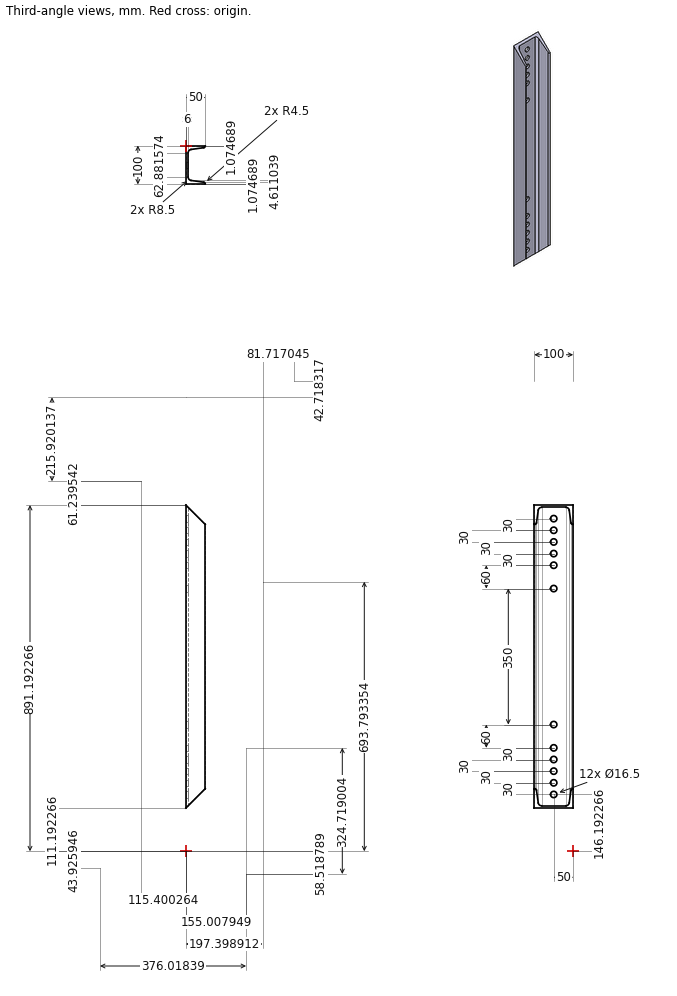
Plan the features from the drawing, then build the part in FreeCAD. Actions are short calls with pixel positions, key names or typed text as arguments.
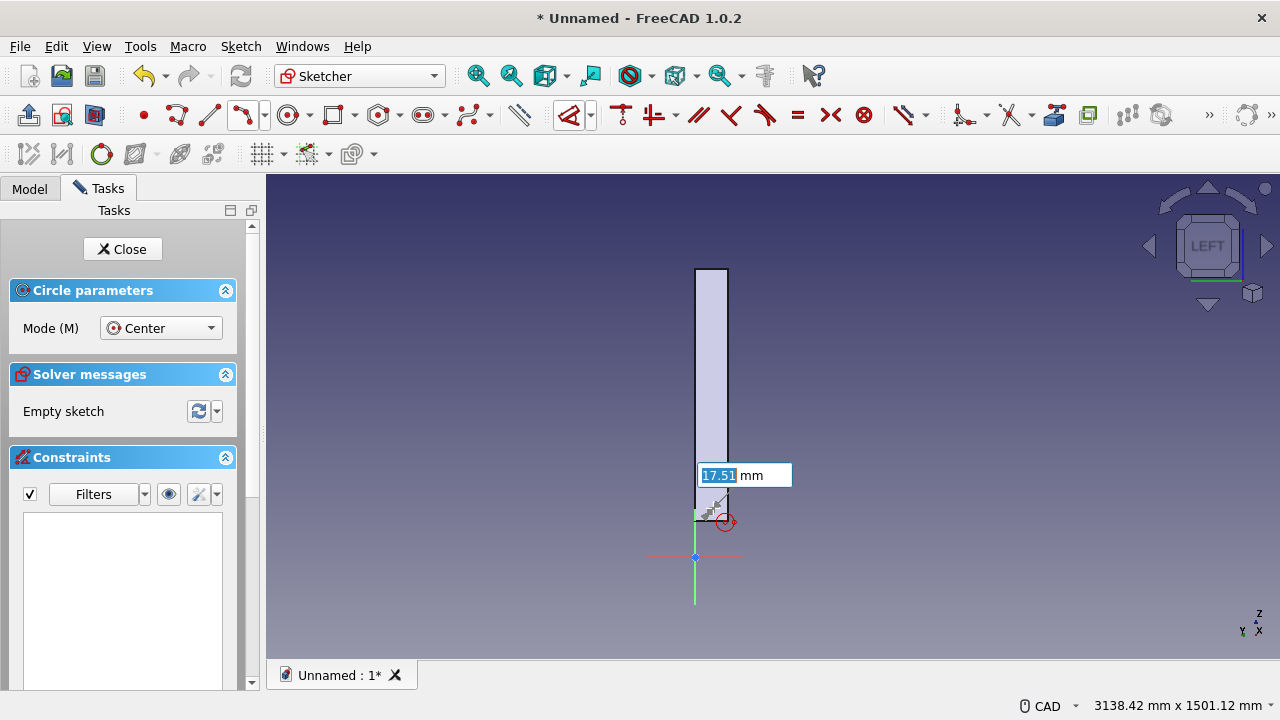
text(16.5)
key(Return)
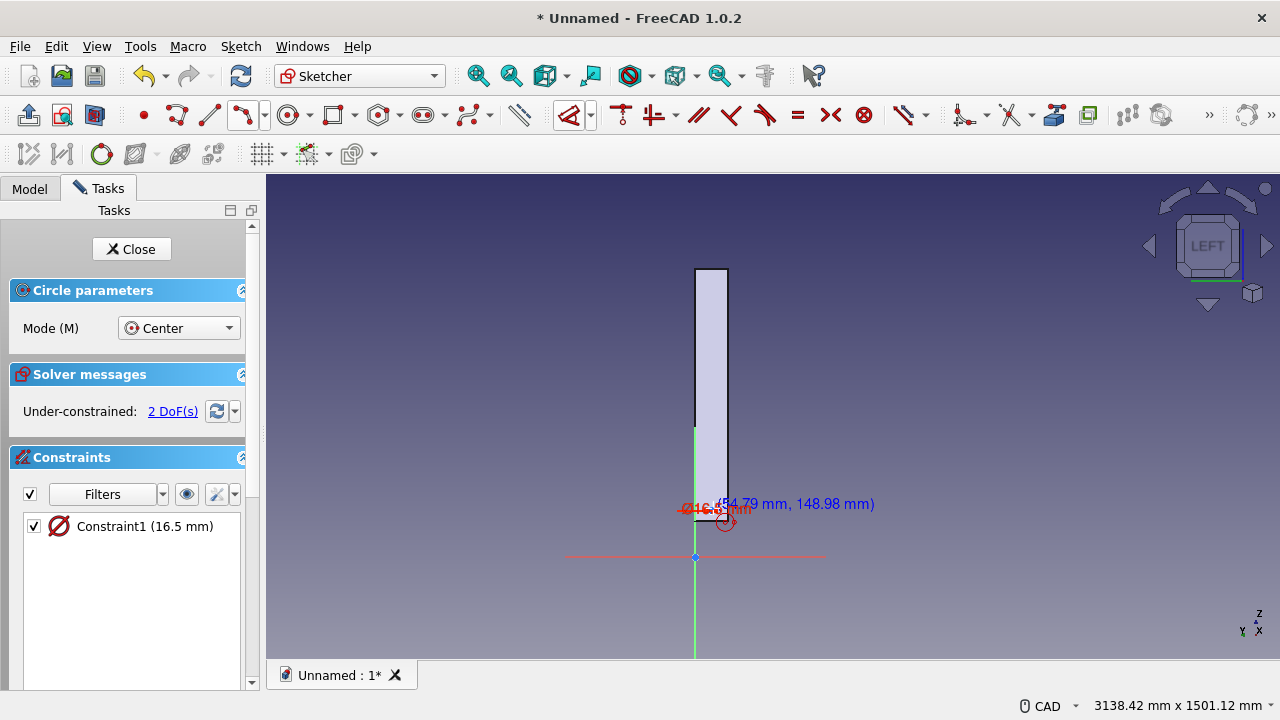
scroll(711, 500, up, 11)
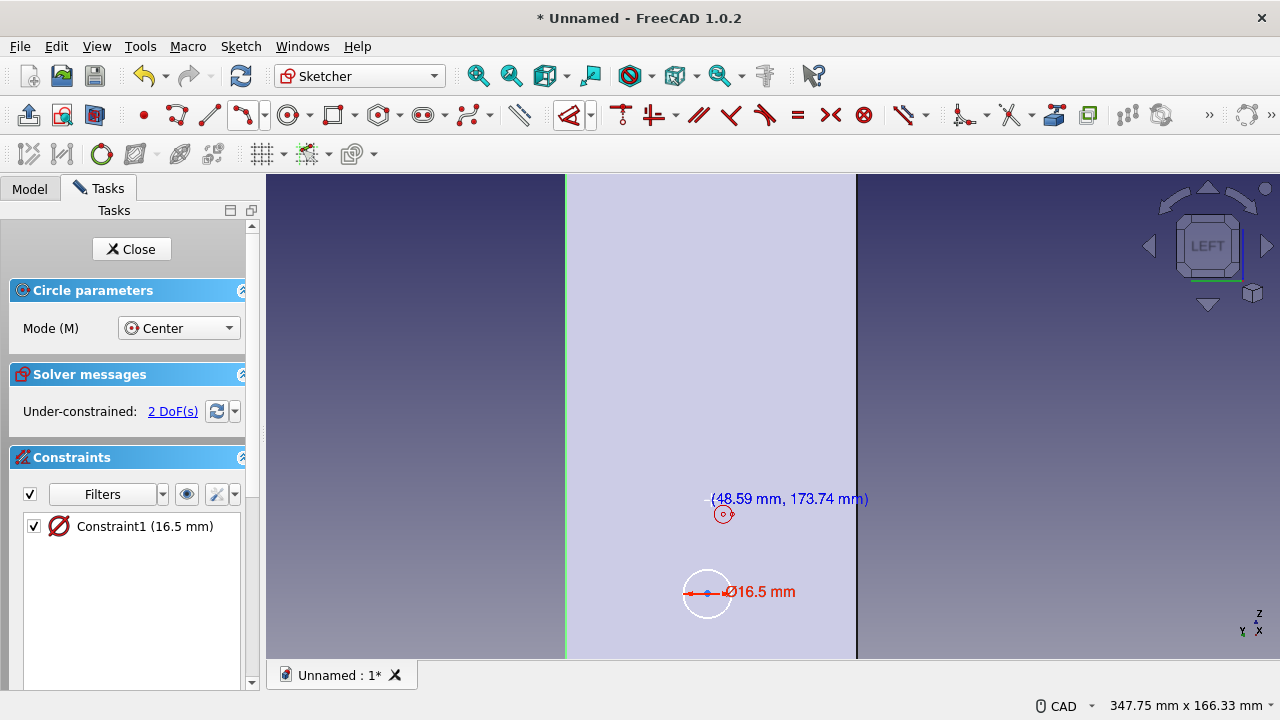
scroll(711, 500, down, 11)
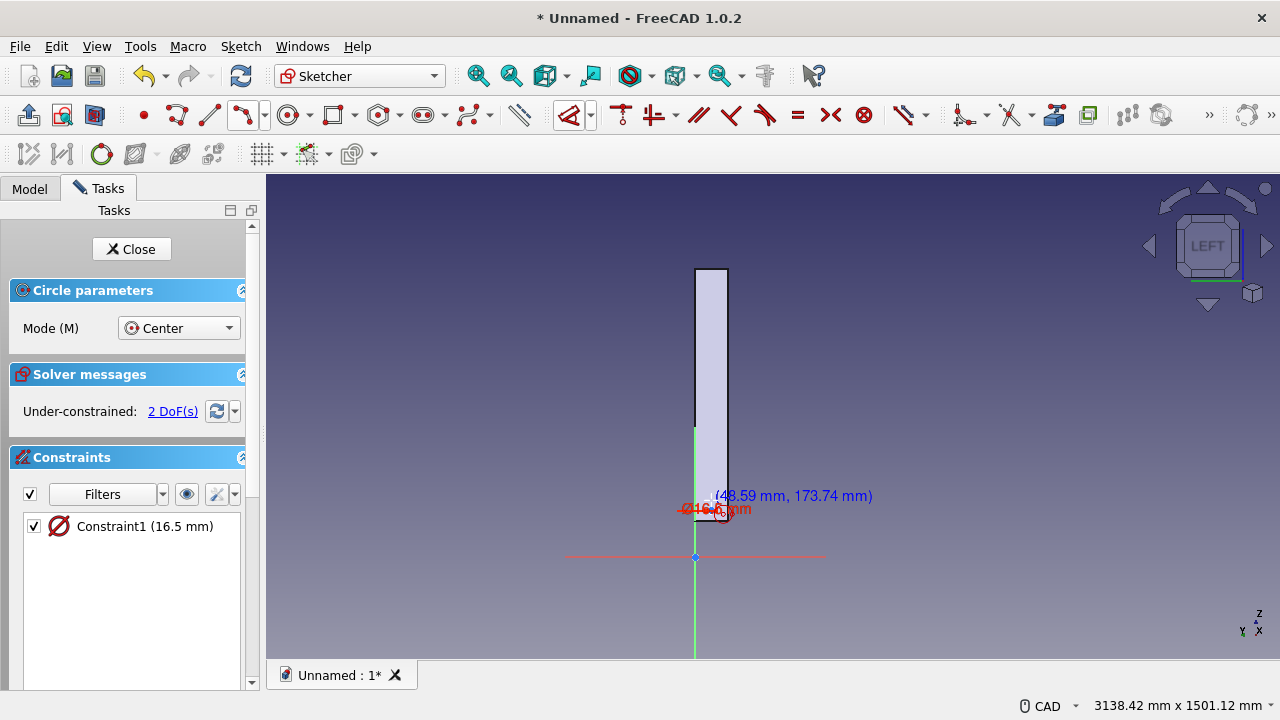
scroll(711, 500, up, 5)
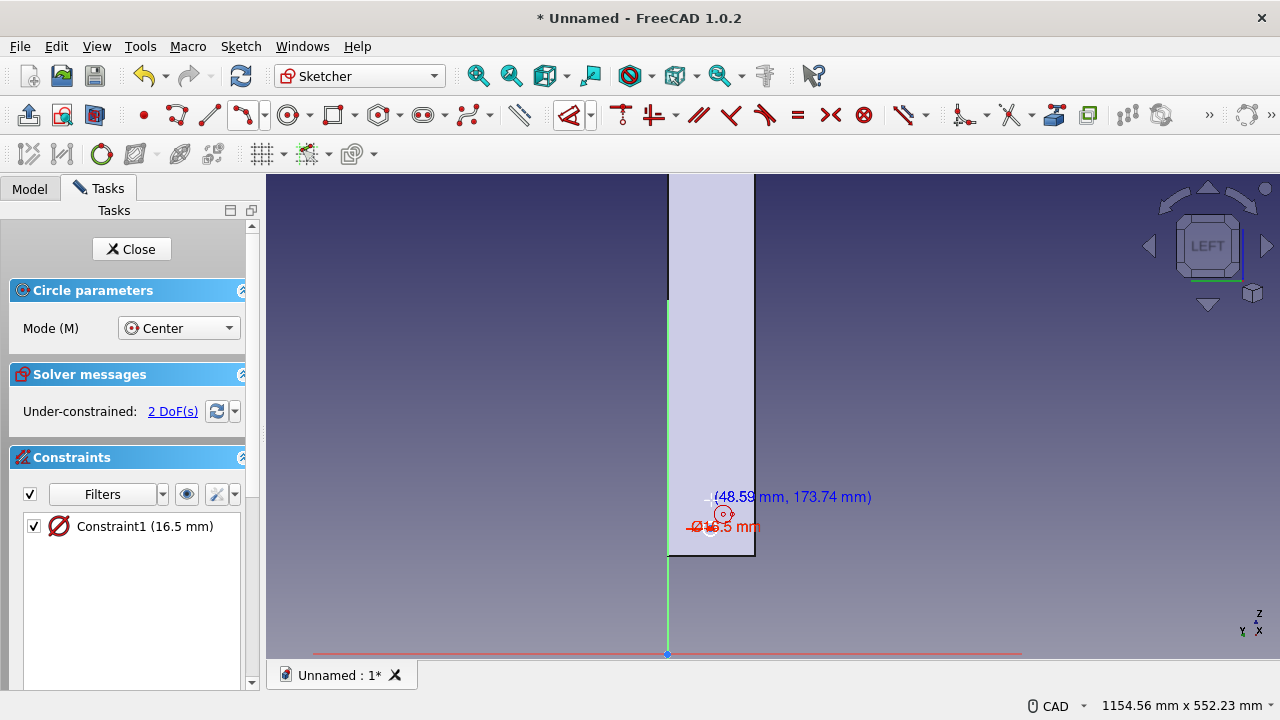
click(711, 499)
move(717, 494)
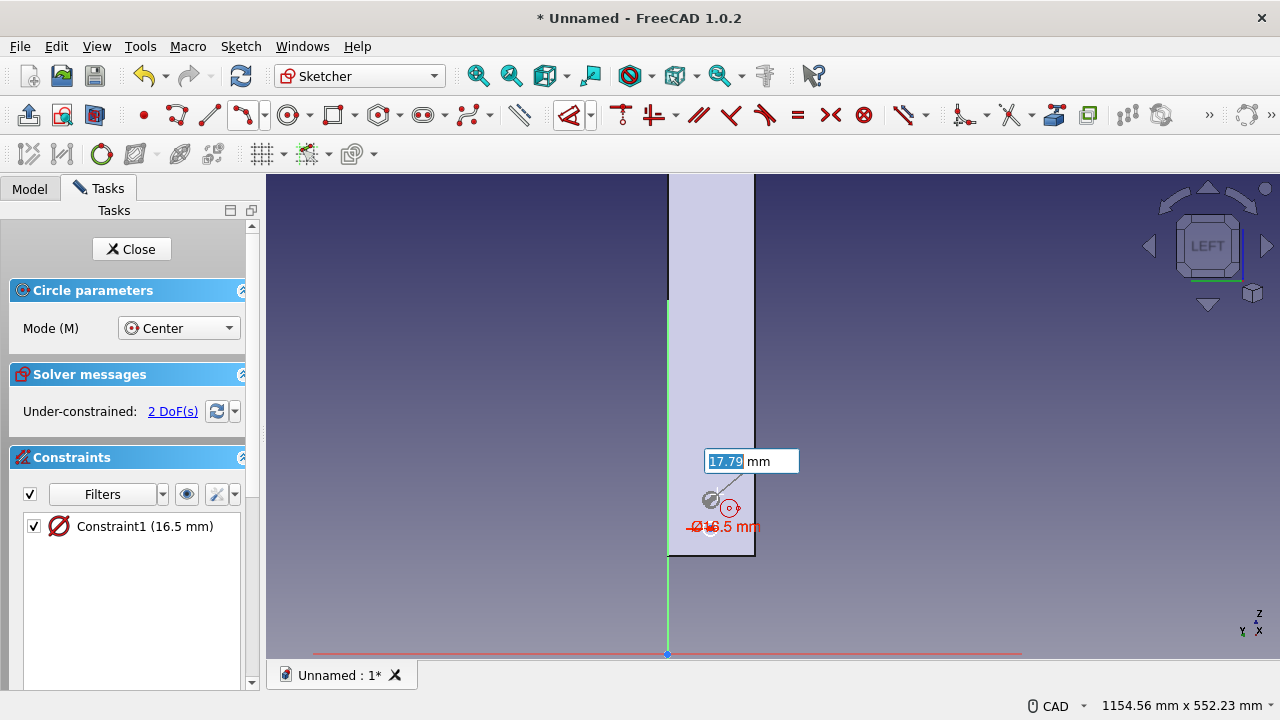
text(16.5)
key(Return)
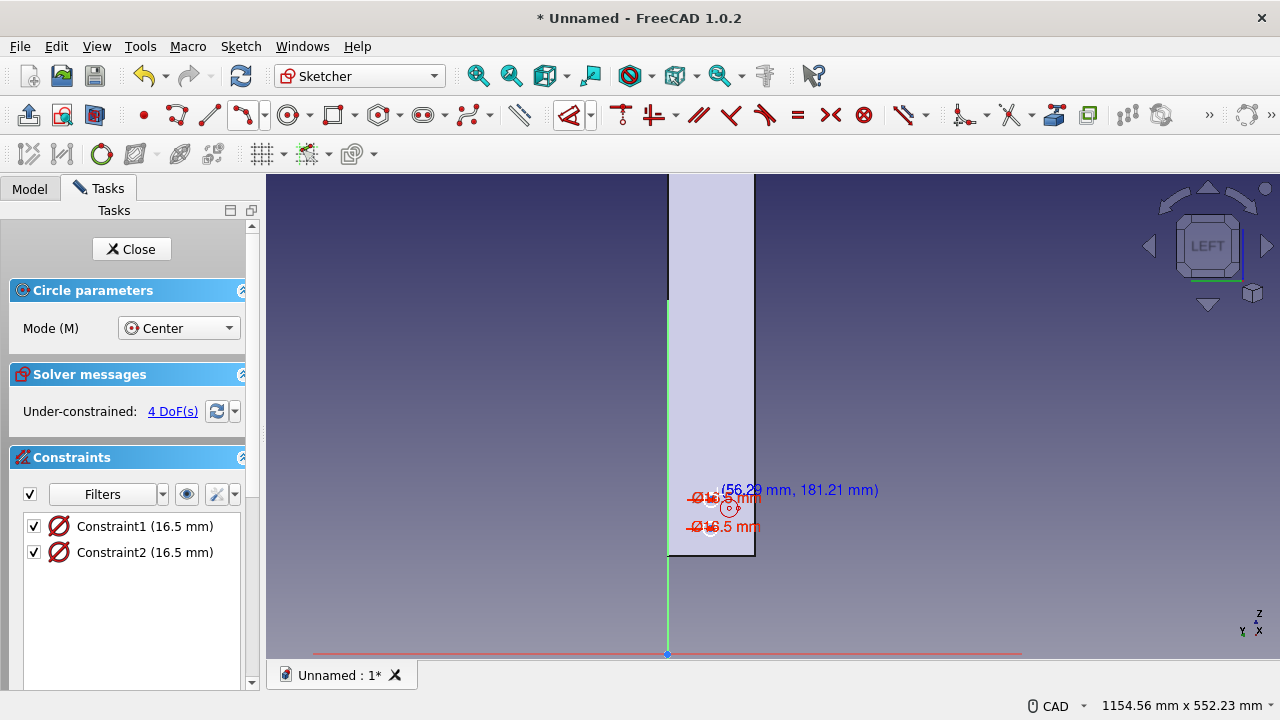
scroll(711, 473, up, 6)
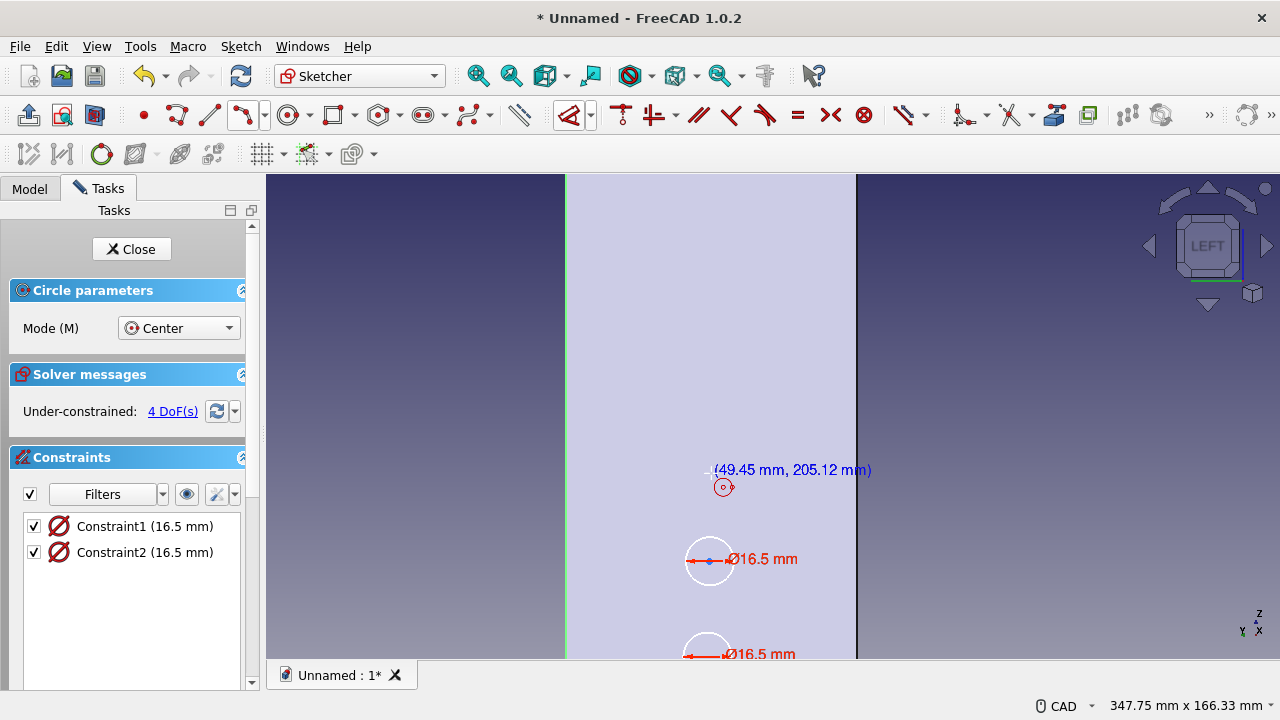
scroll(711, 492, down, 11)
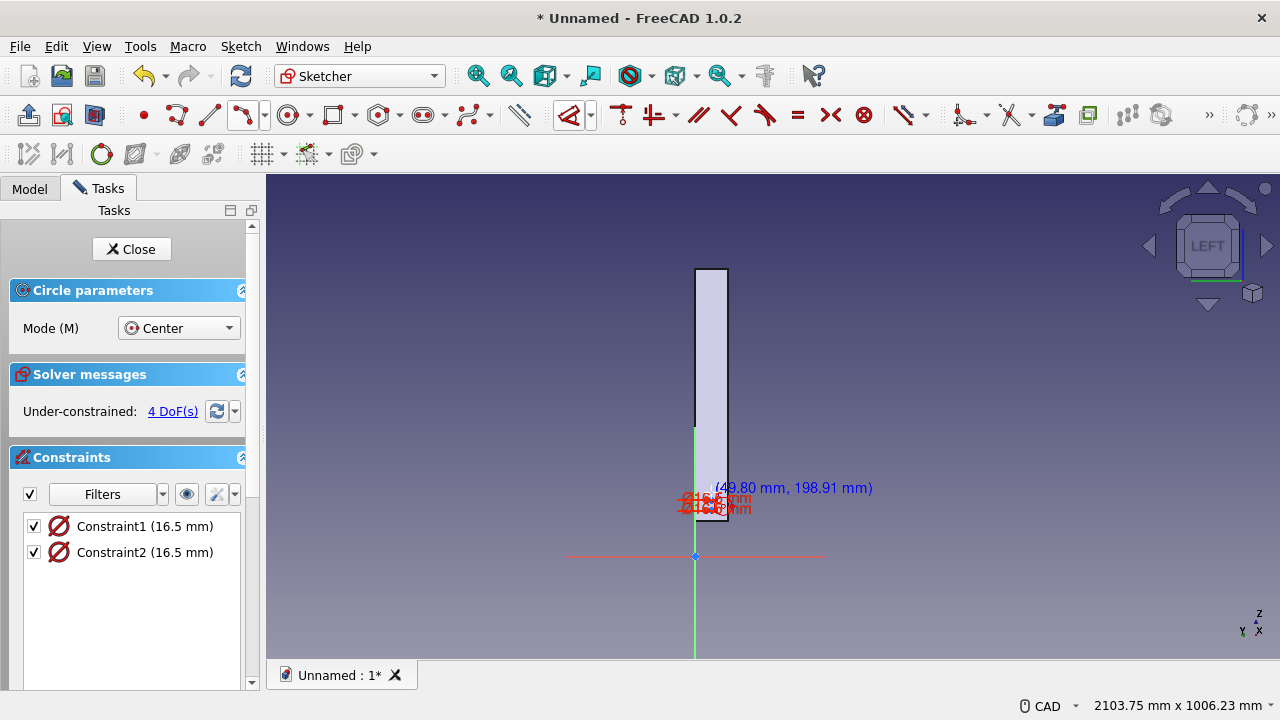
scroll(711, 490, up, 5)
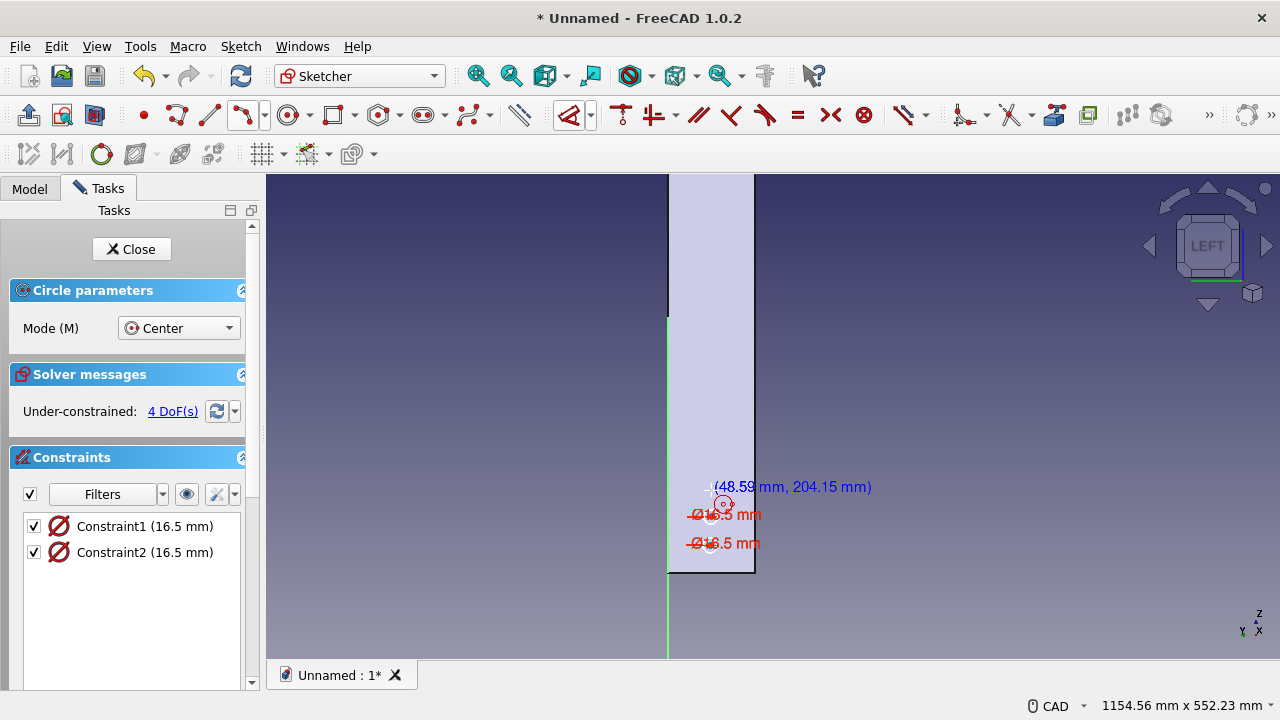
click(711, 490)
move(717, 485)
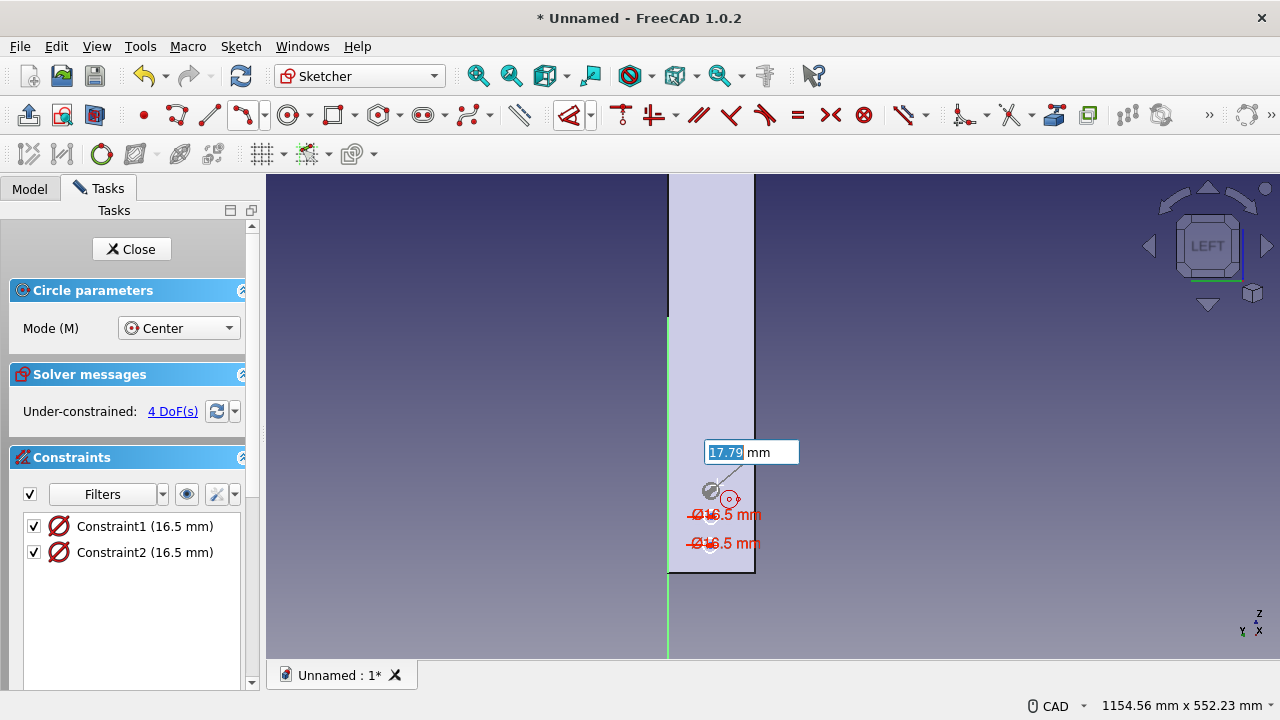
text(16.5)
key(Return)